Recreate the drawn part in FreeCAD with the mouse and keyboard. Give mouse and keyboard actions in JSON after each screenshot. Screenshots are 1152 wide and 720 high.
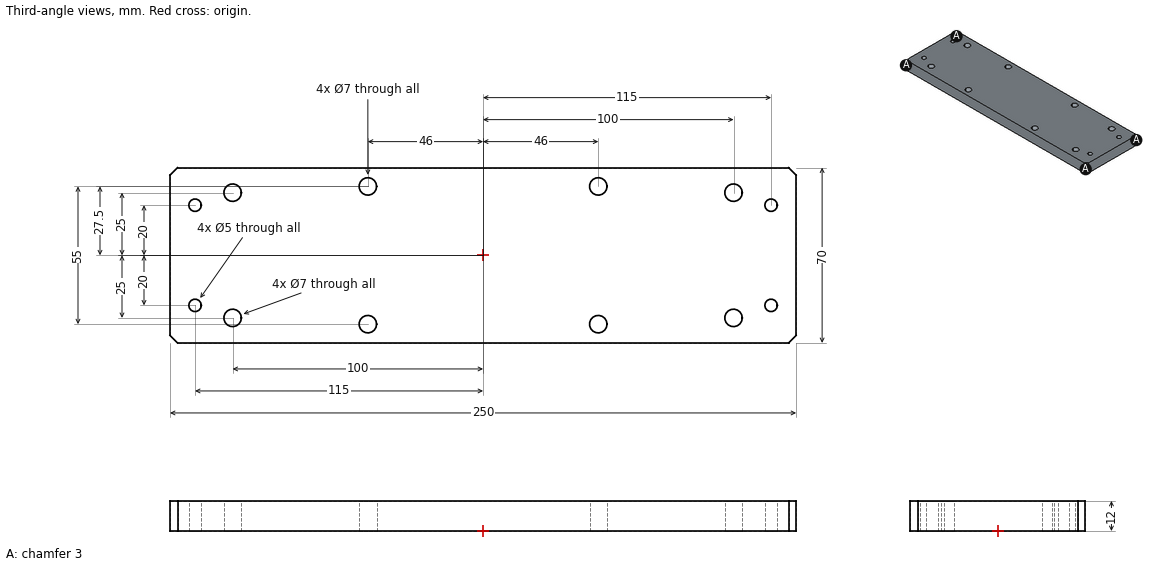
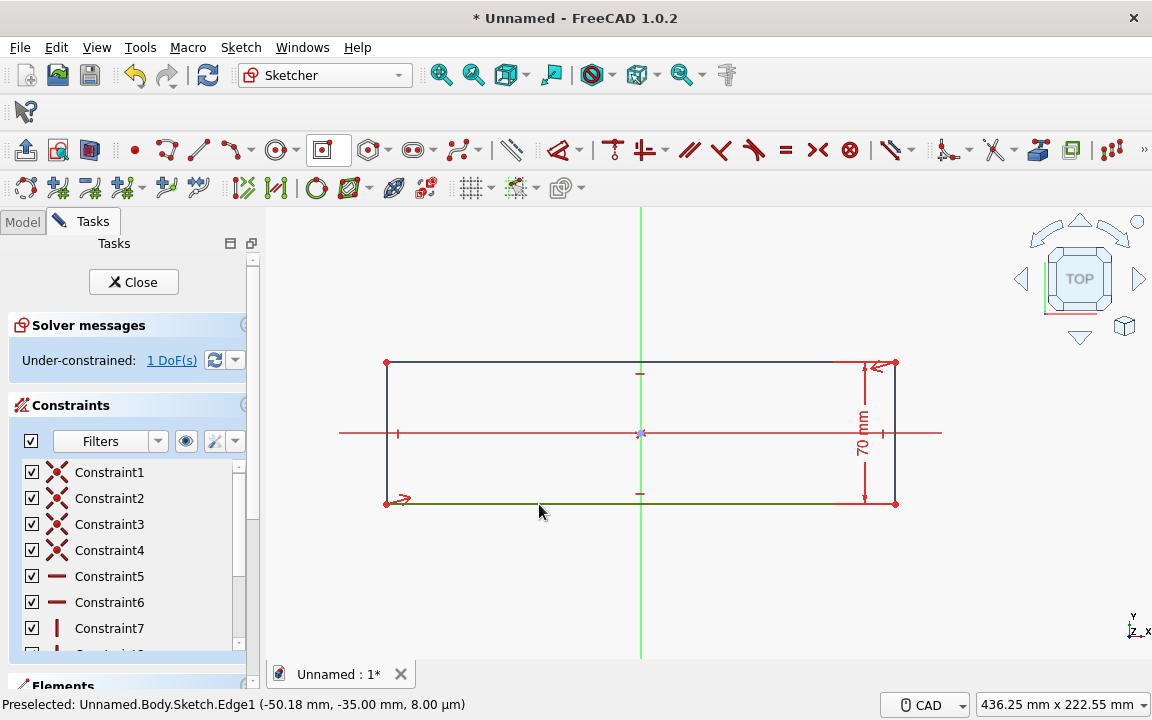
{"action": "key", "text": "l"}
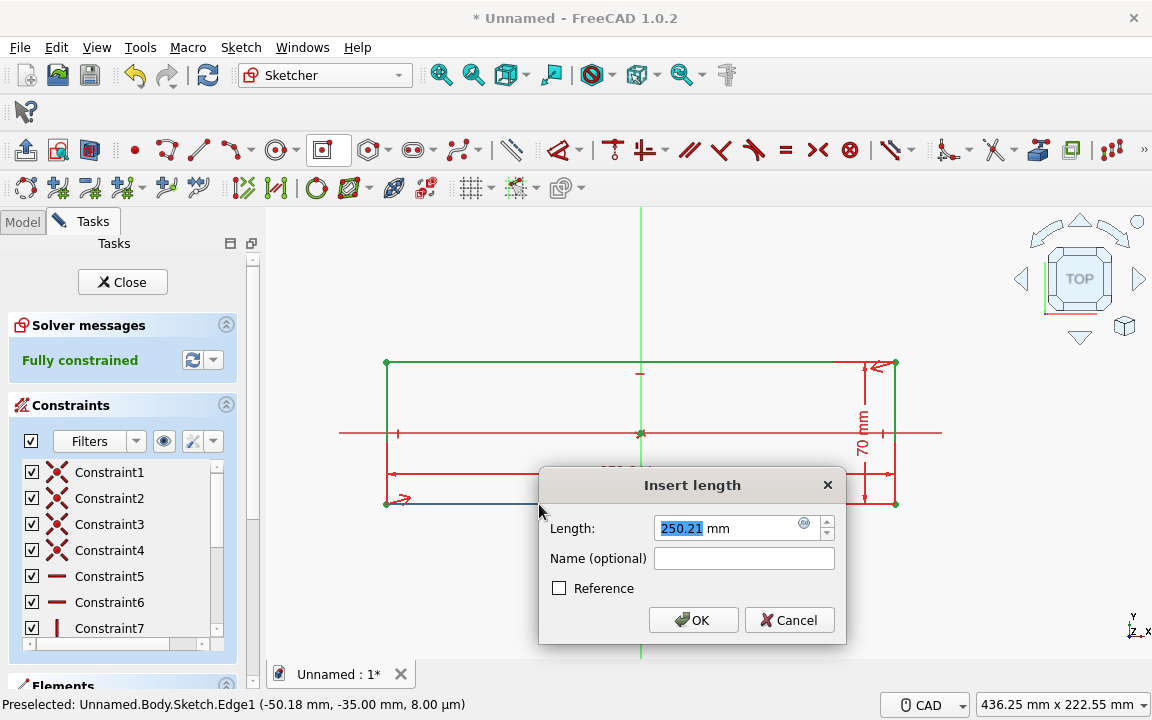
{"action": "type", "text": "250"}
{"action": "key", "text": "Return"}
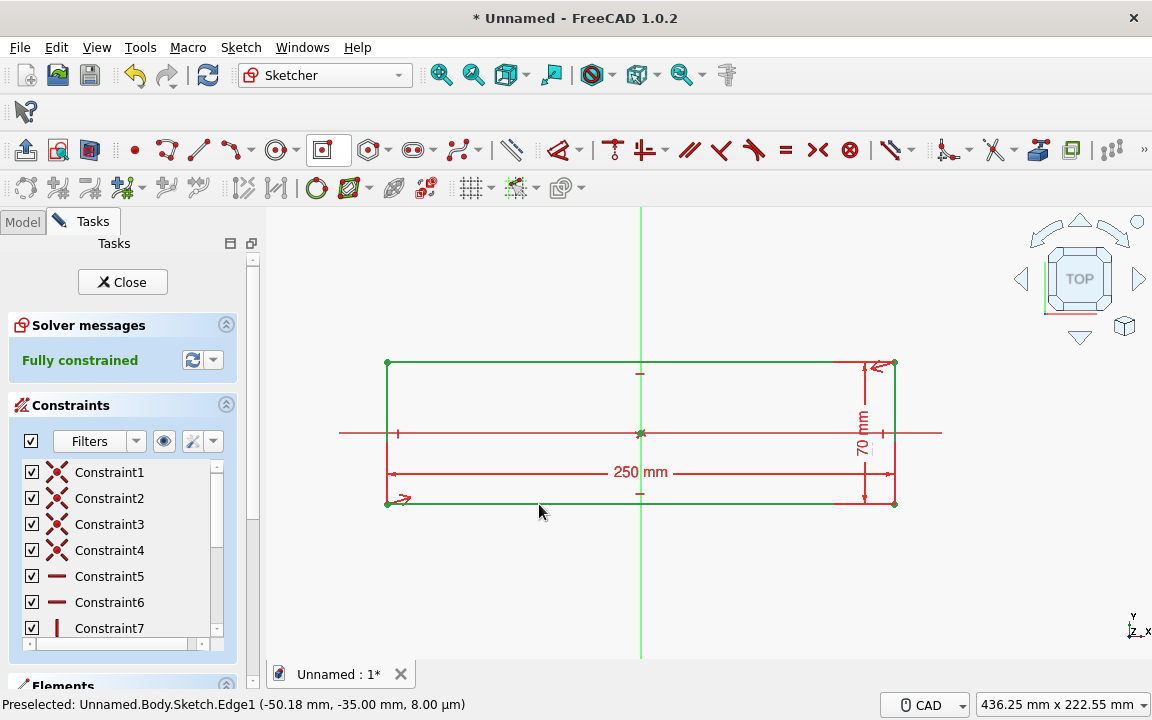
{"action": "left_click", "coordinate": [123, 282]}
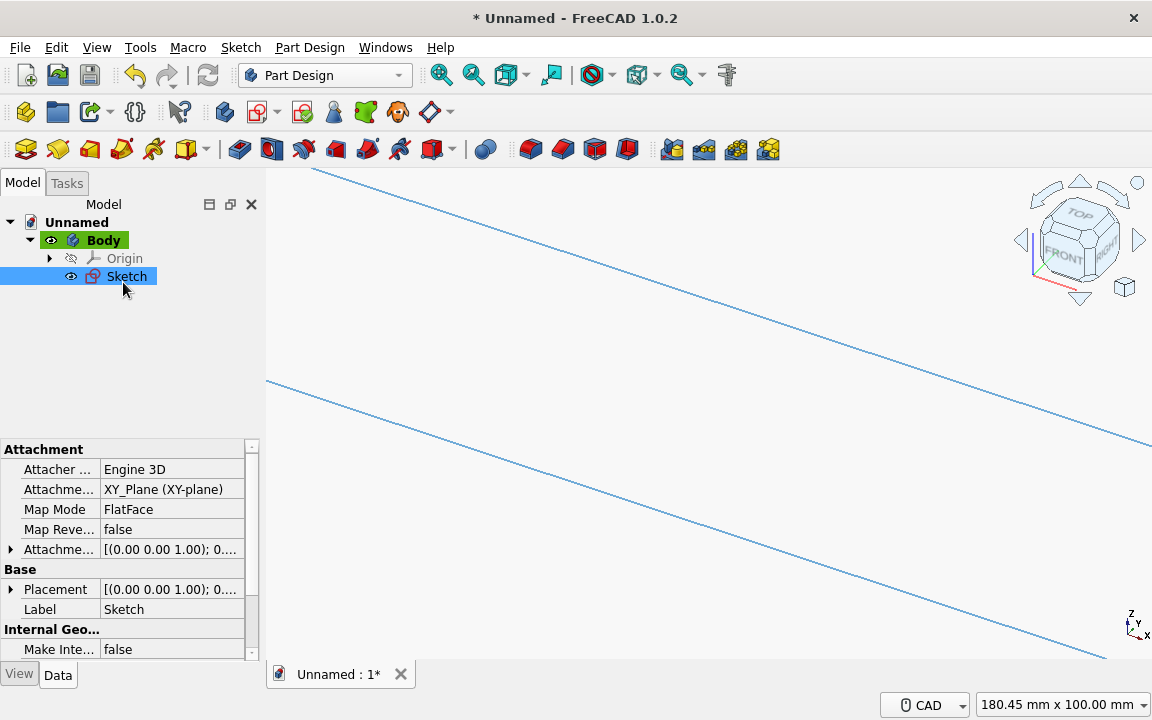
{"action": "left_click", "coordinate": [26, 150]}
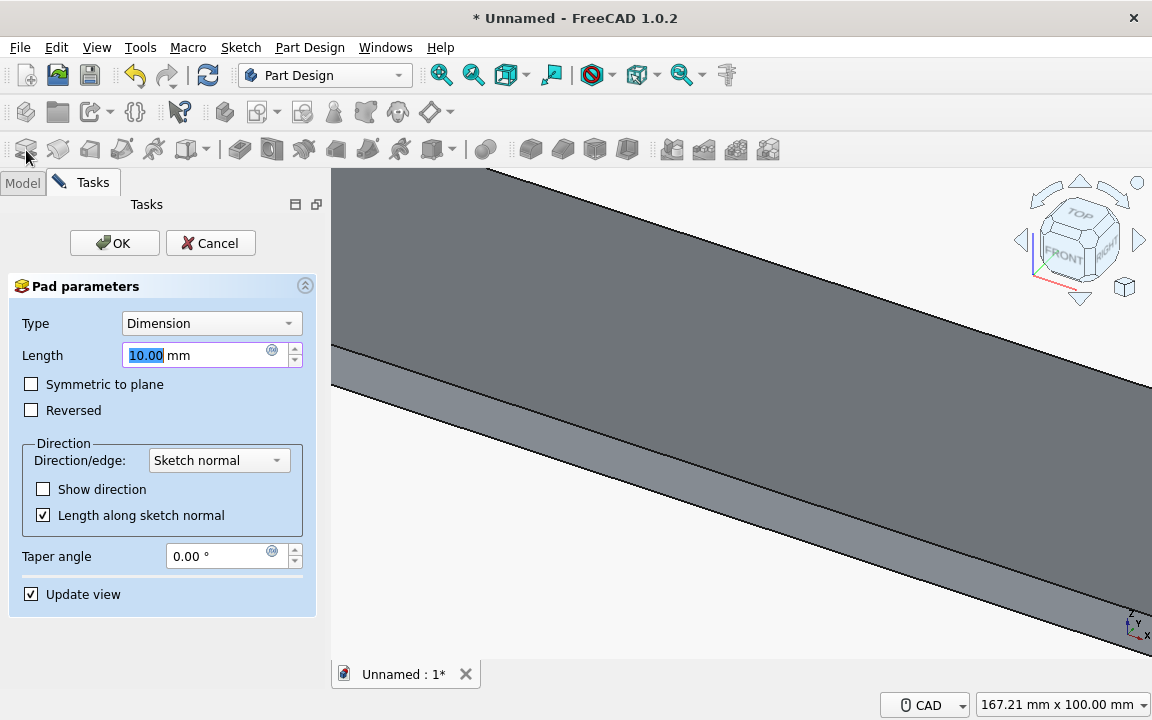
{"action": "type", "text": "12"}
{"action": "key", "text": "Tab"}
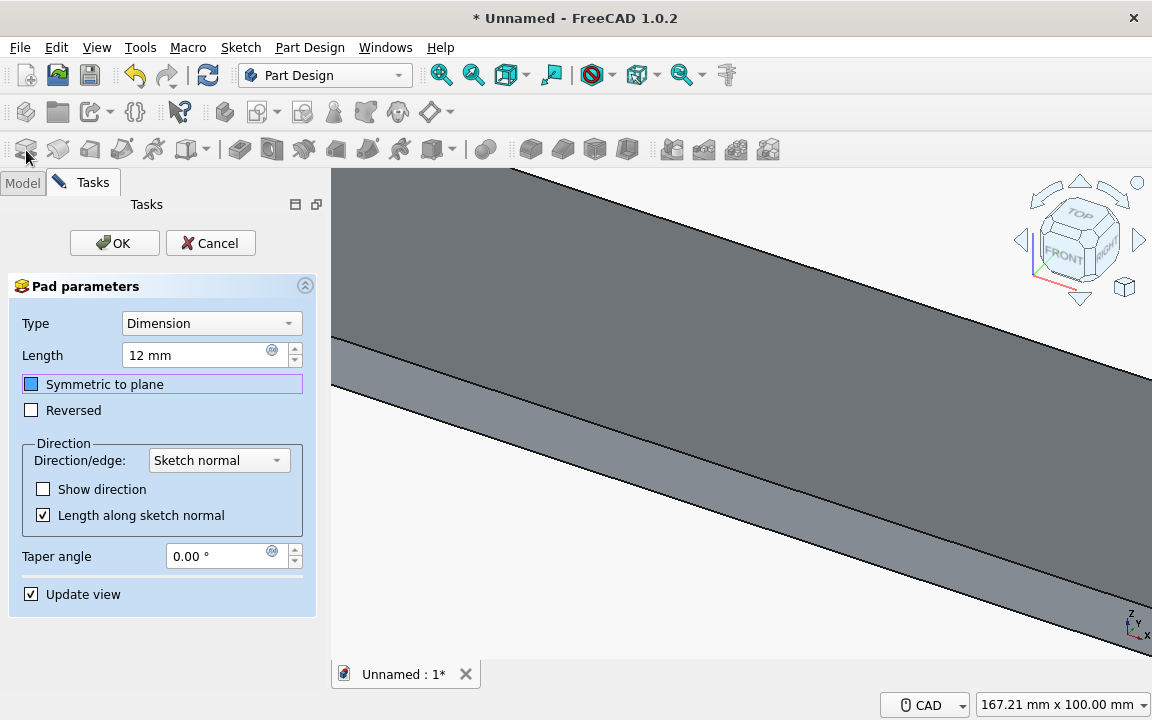
{"action": "left_click", "coordinate": [115, 243]}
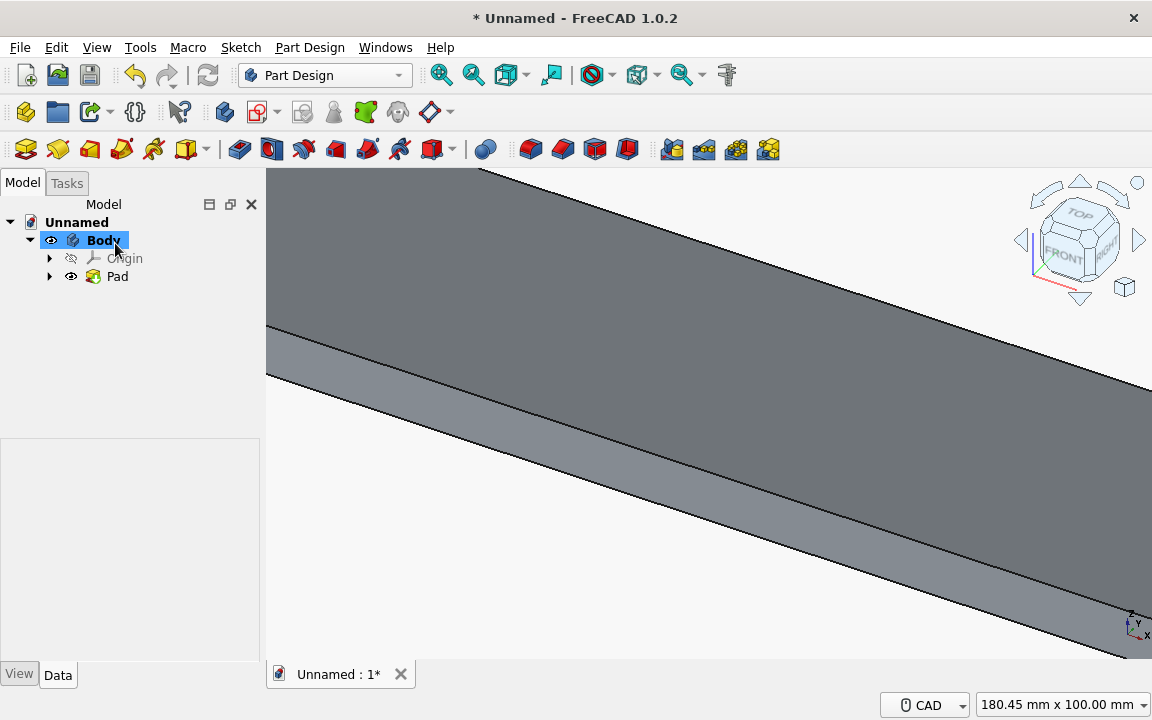
{"action": "left_click", "coordinate": [442, 76]}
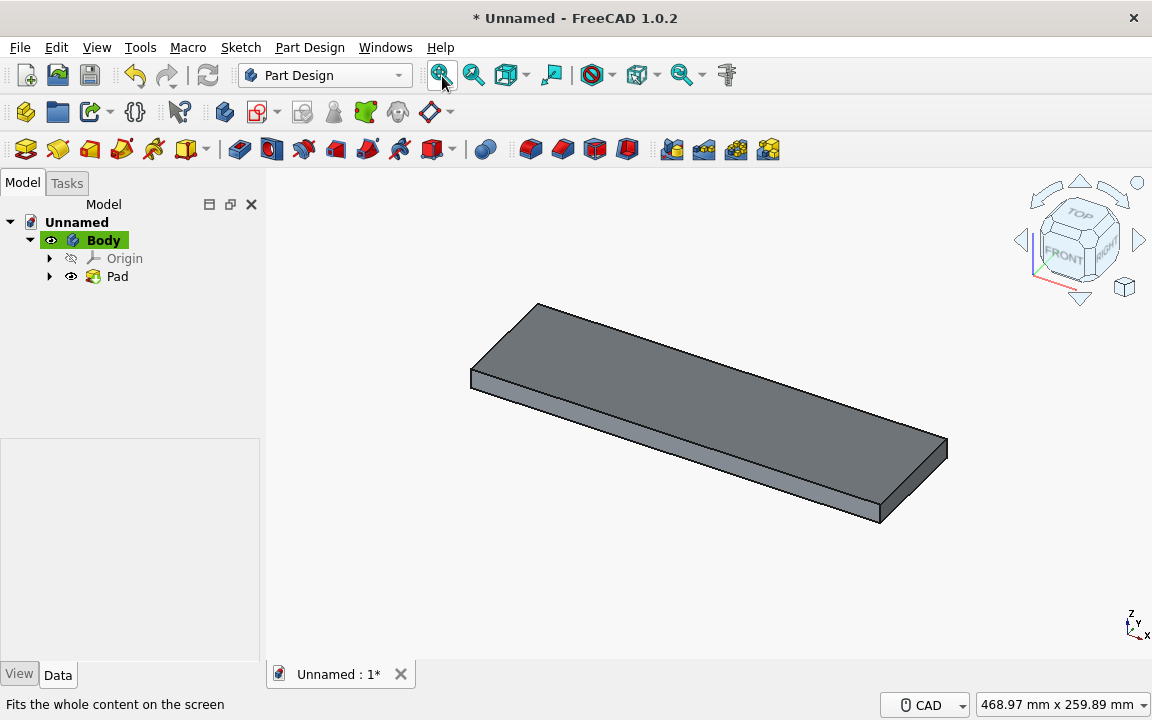
{"action": "left_click", "coordinate": [880, 513]}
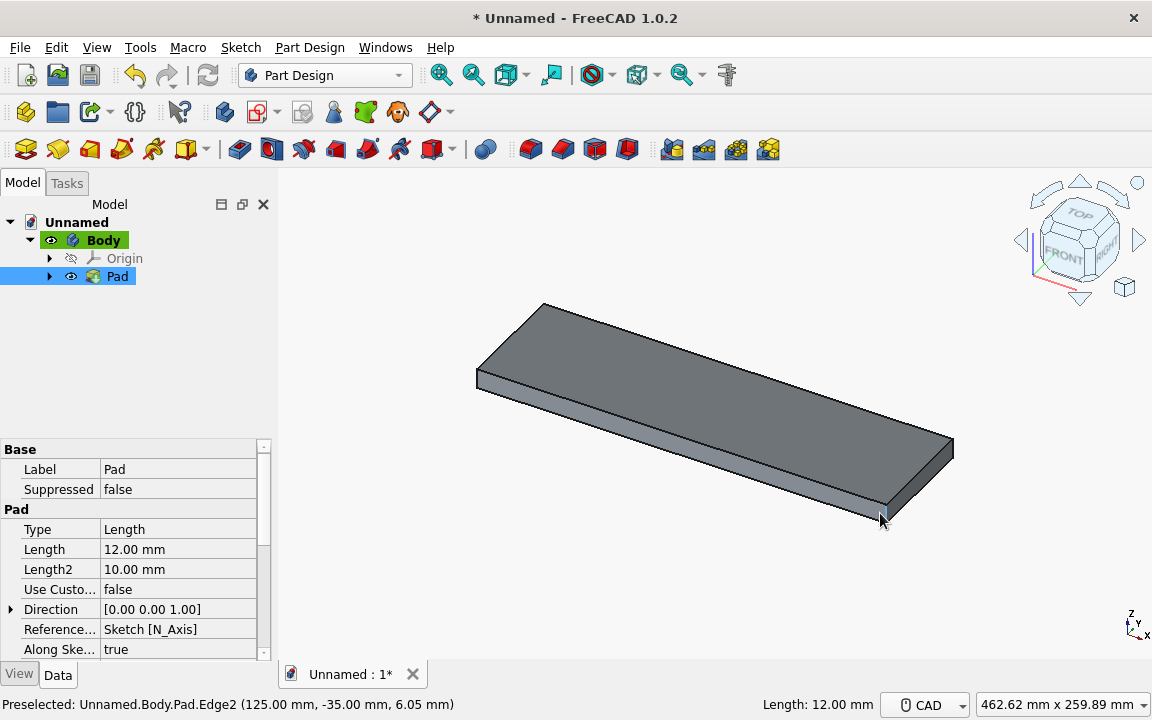
{"action": "key", "text": "0"}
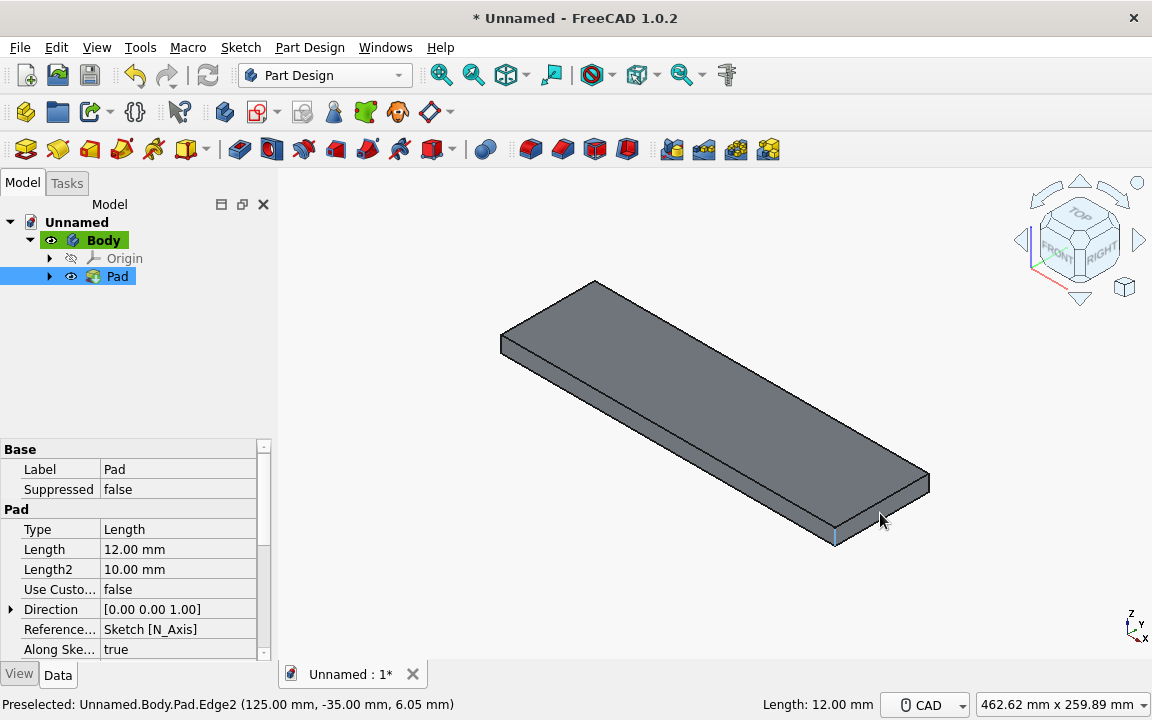
{"action": "key", "text": "2"}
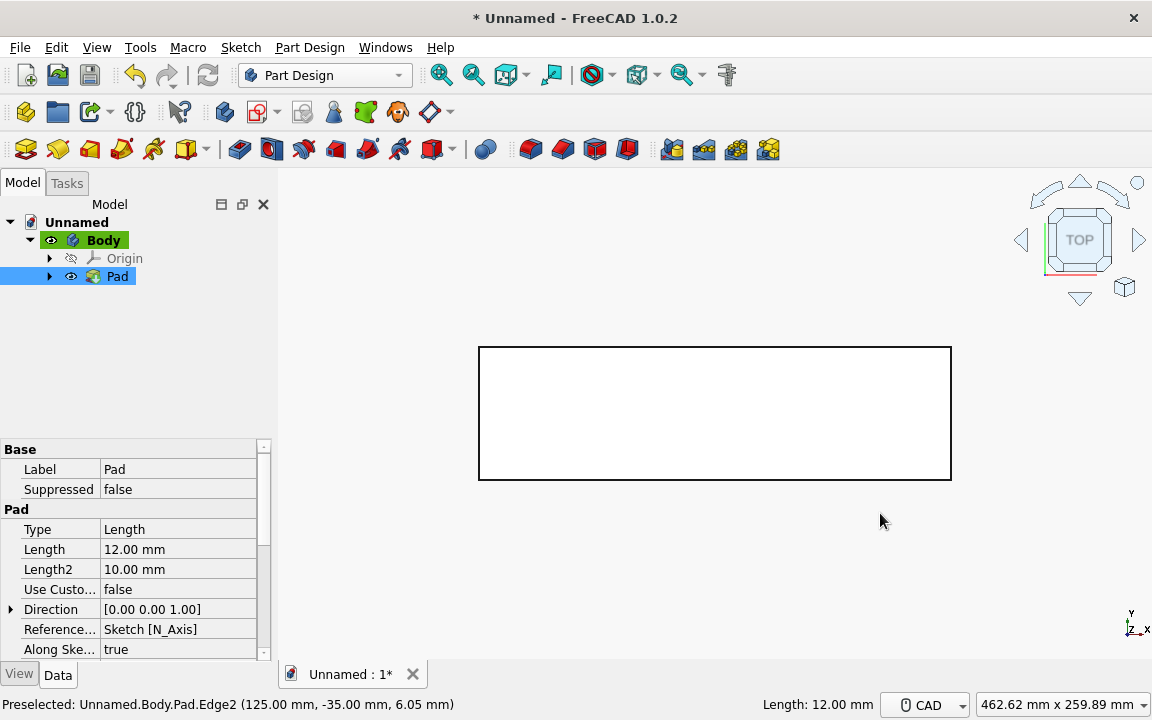
{"action": "key", "text": "1"}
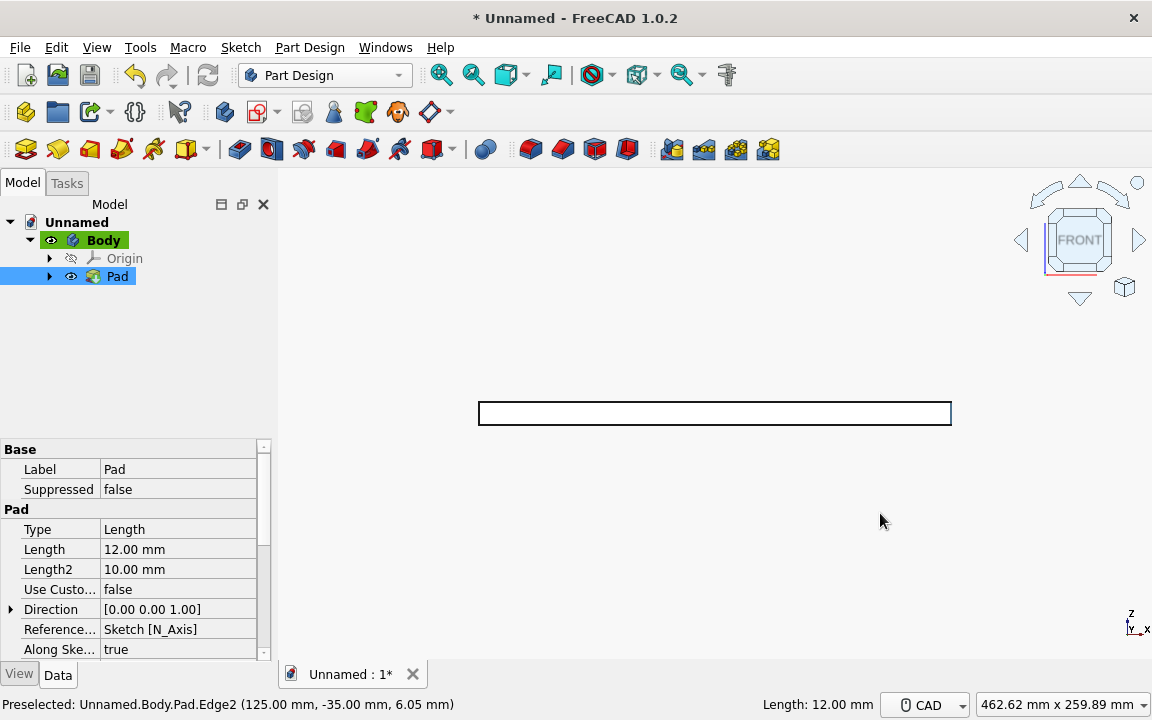
{"action": "left_click", "coordinate": [479, 412], "text": "ctrl"}